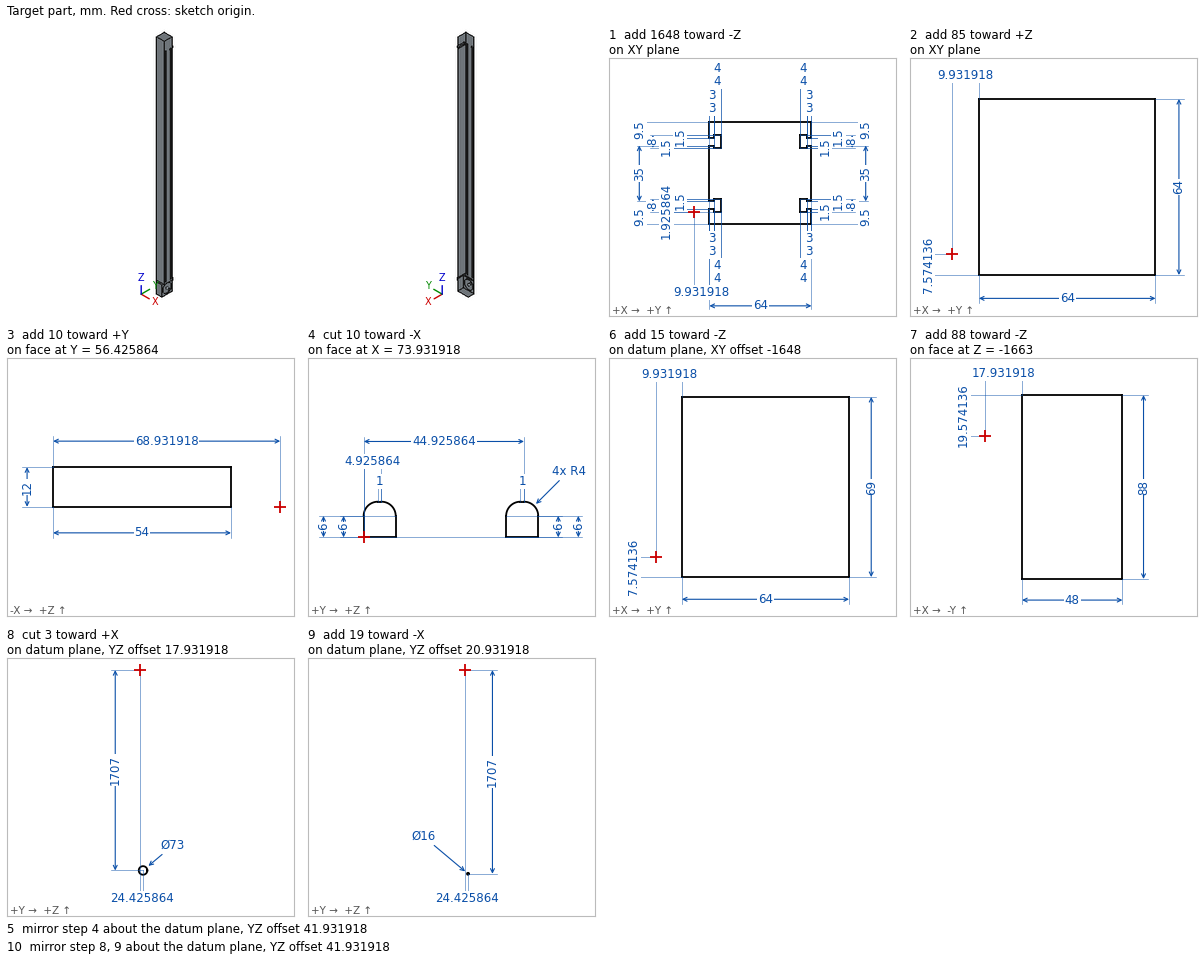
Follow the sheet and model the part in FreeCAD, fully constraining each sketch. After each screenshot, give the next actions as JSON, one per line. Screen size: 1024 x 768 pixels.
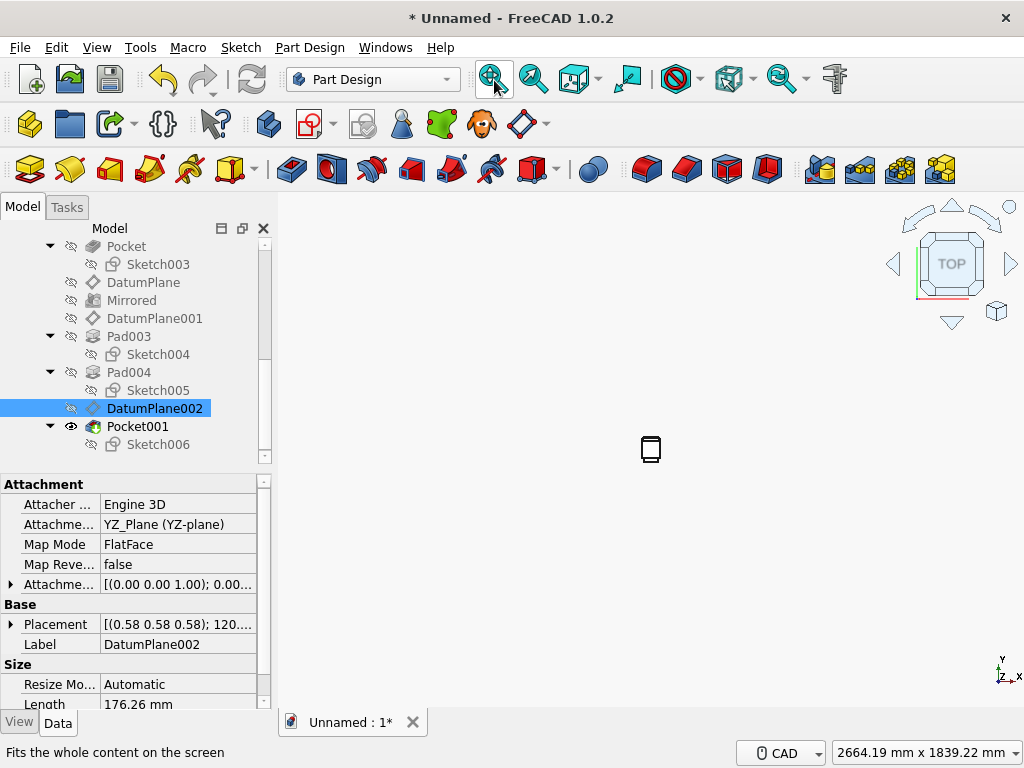
{"action": "key", "text": "1"}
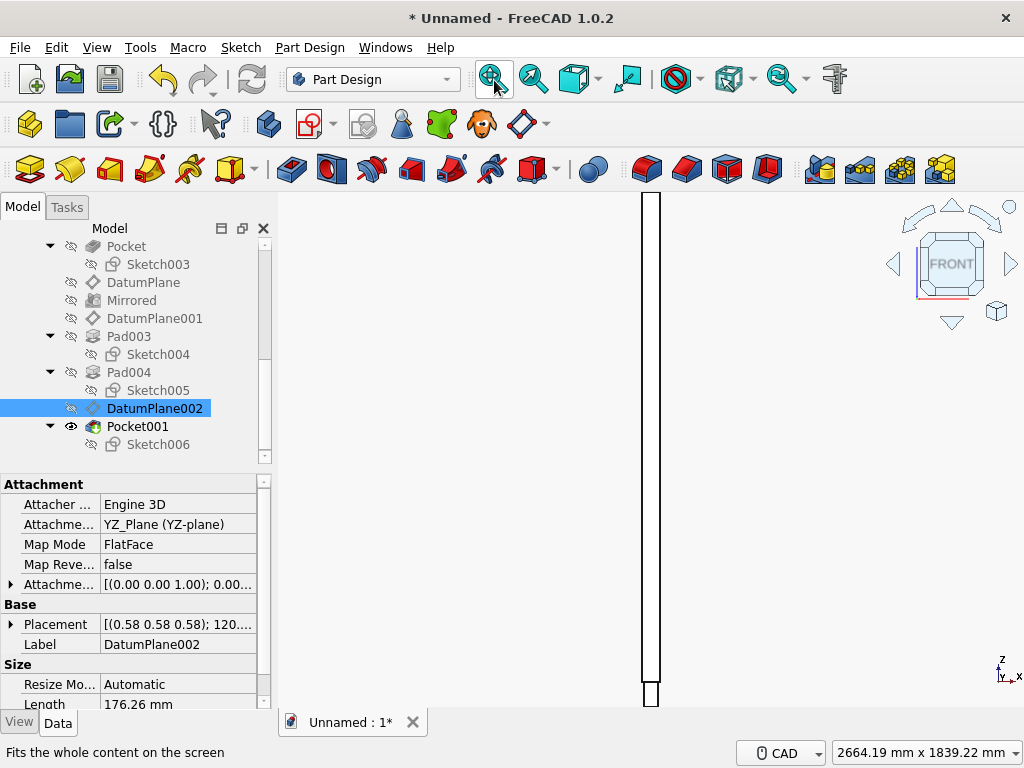
{"action": "left_click", "coordinate": [494, 80]}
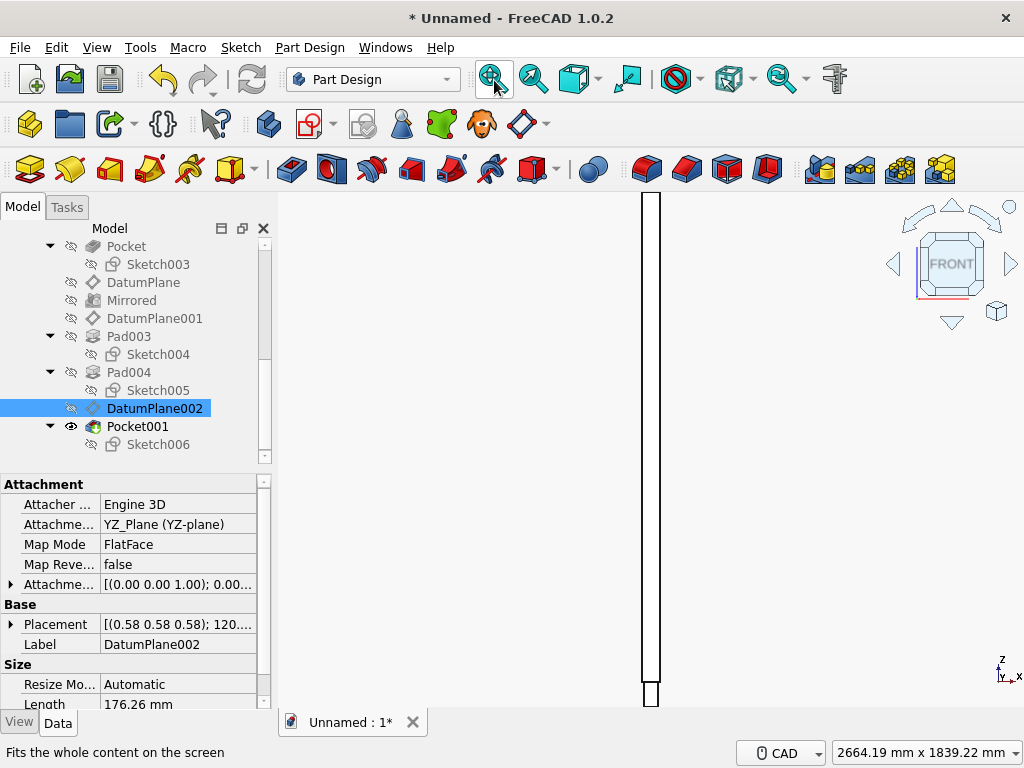
{"action": "scroll", "coordinate": [140, 350], "scroll_direction": "down", "scroll_amount": 3}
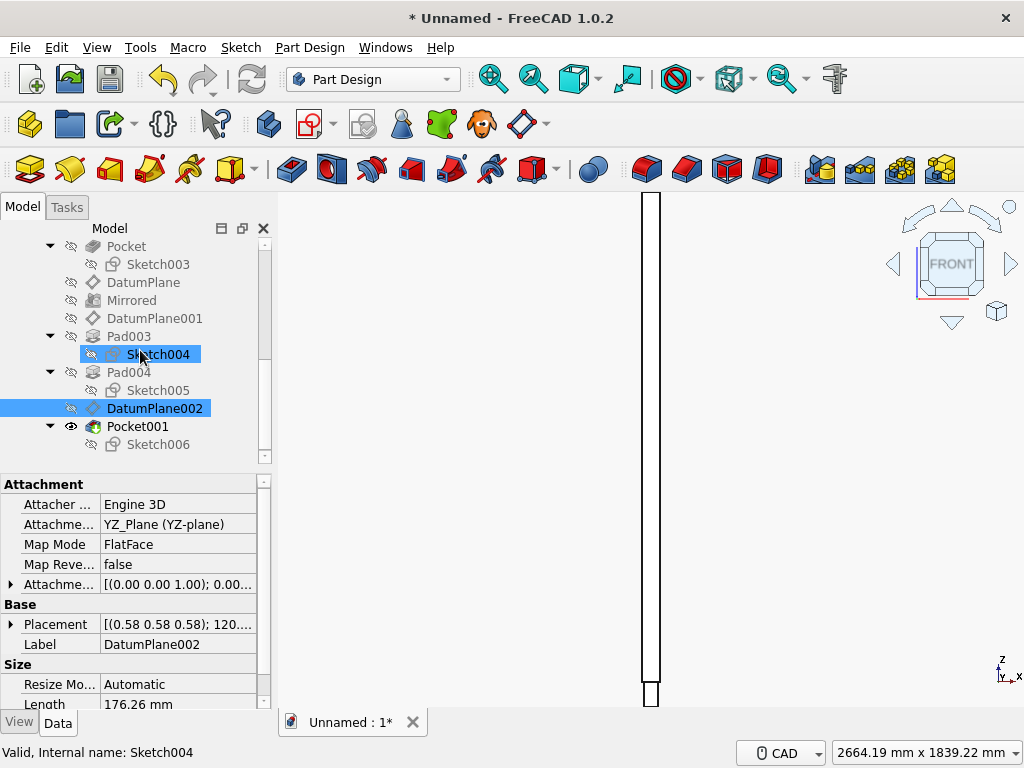
{"action": "scroll", "coordinate": [140, 350], "scroll_direction": "up", "scroll_amount": 15}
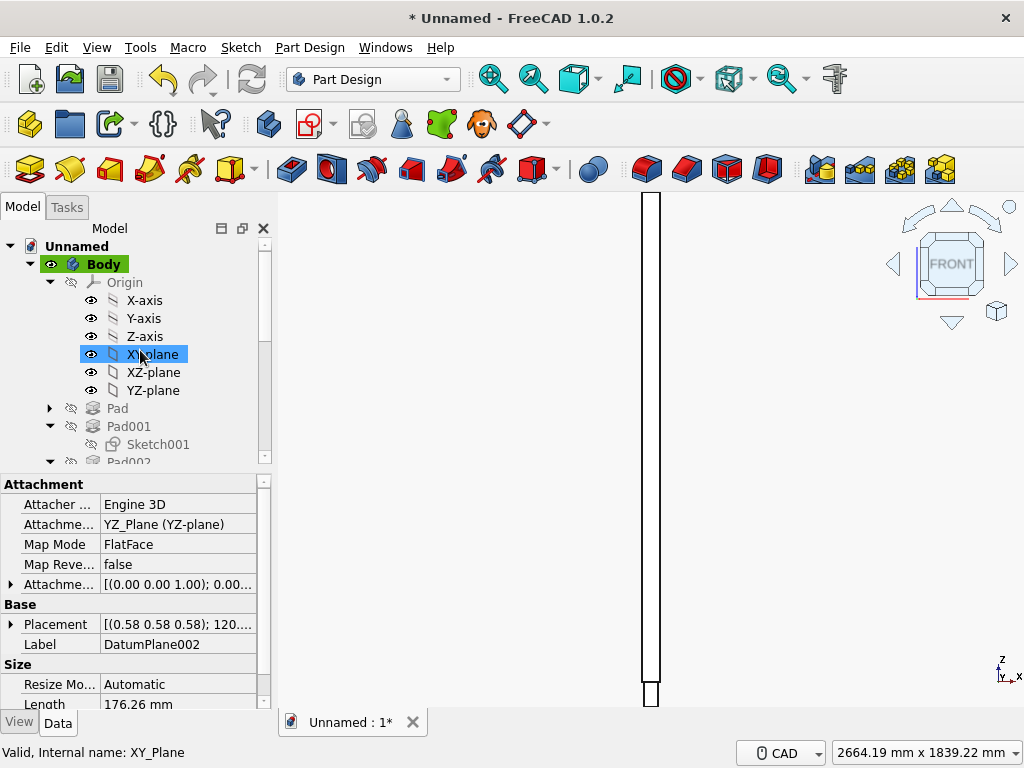
{"action": "left_click", "coordinate": [136, 390]}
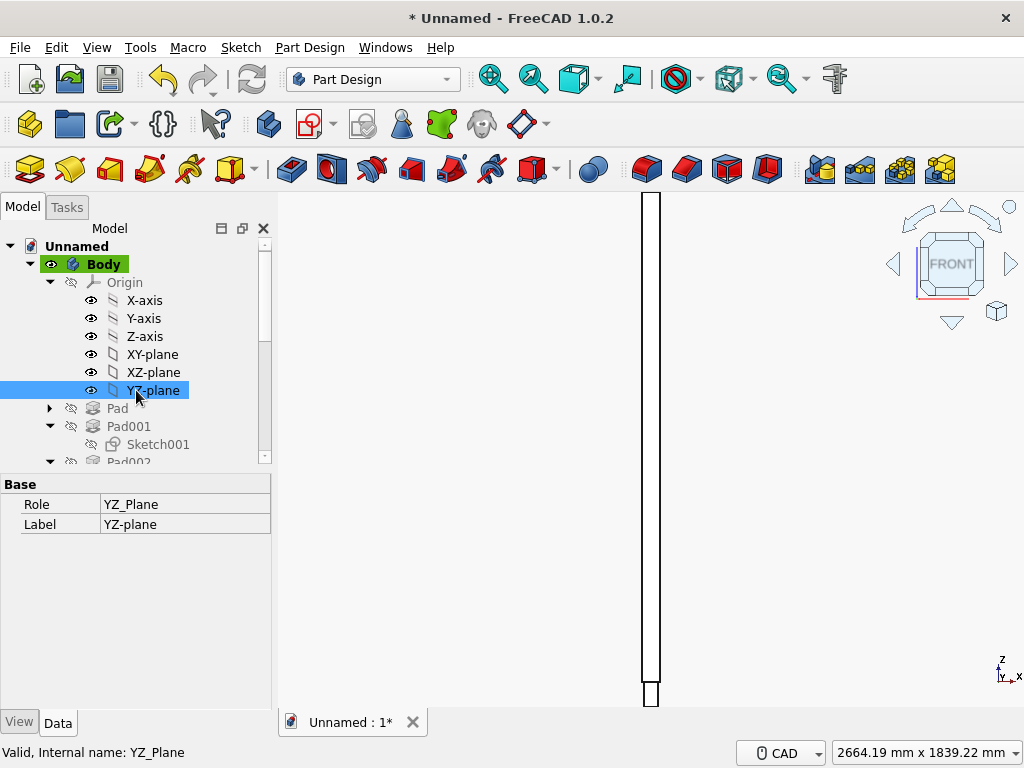
{"action": "left_click", "coordinate": [522, 124]}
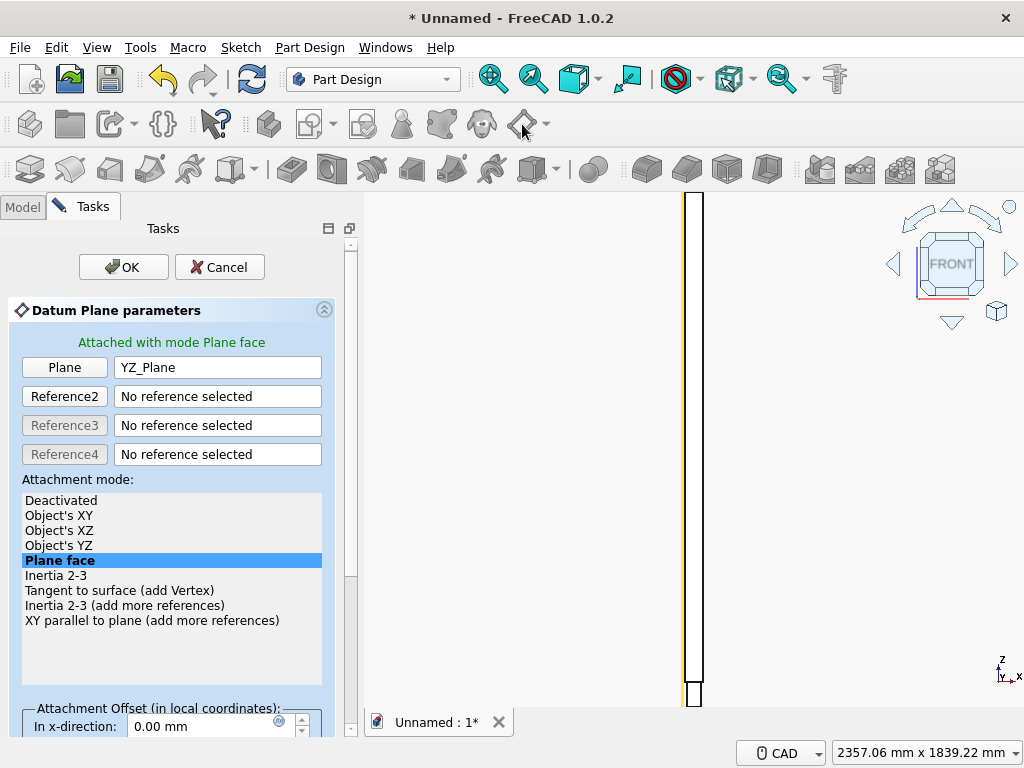
{"action": "scroll", "coordinate": [351, 487], "scroll_direction": "down", "scroll_amount": 3}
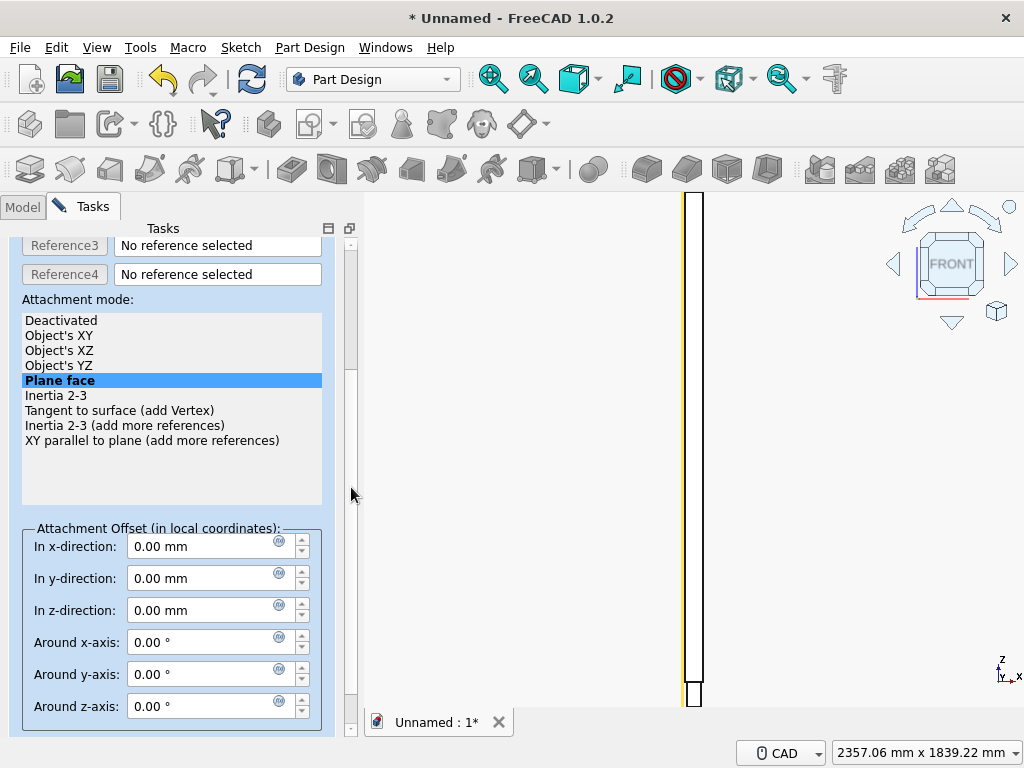
{"action": "triple_click", "coordinate": [210, 610]}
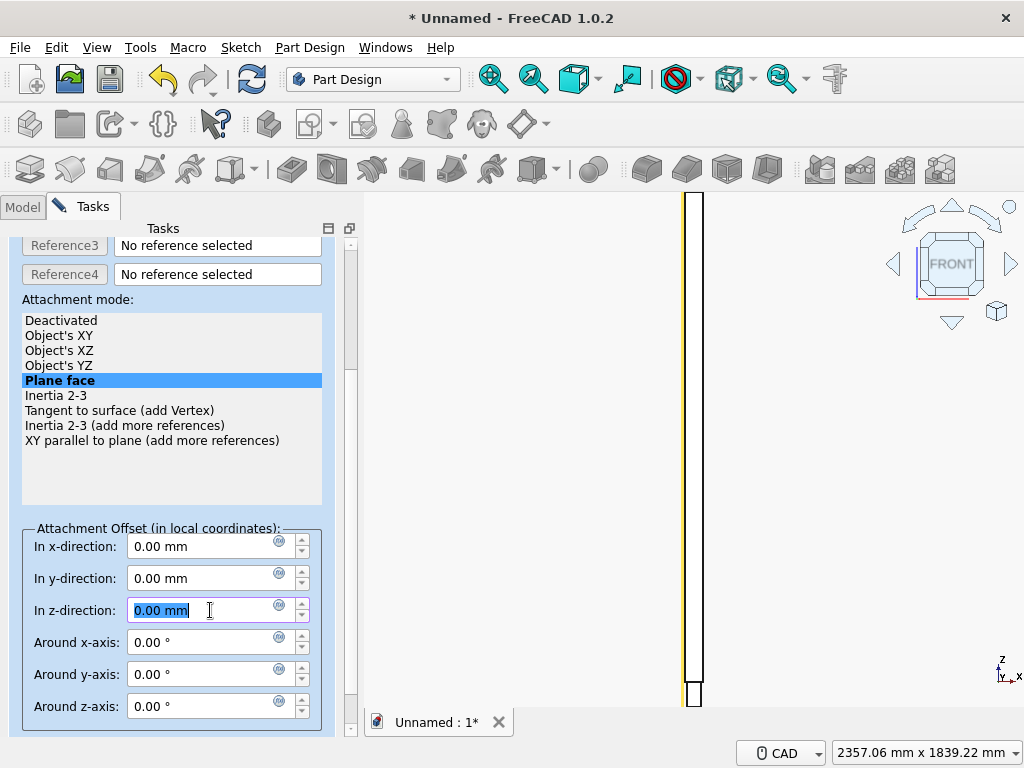
{"action": "type", "text": "20.931918"}
{"action": "key", "text": "Tab"}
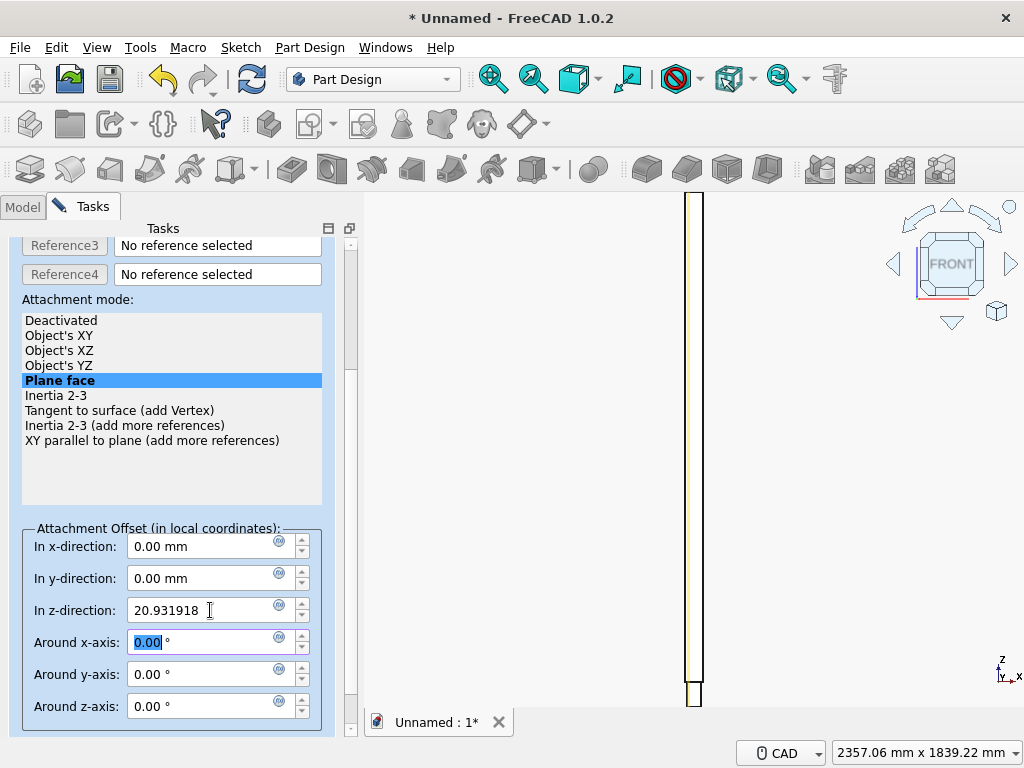
{"action": "scroll", "coordinate": [351, 487], "scroll_direction": "up", "scroll_amount": 4}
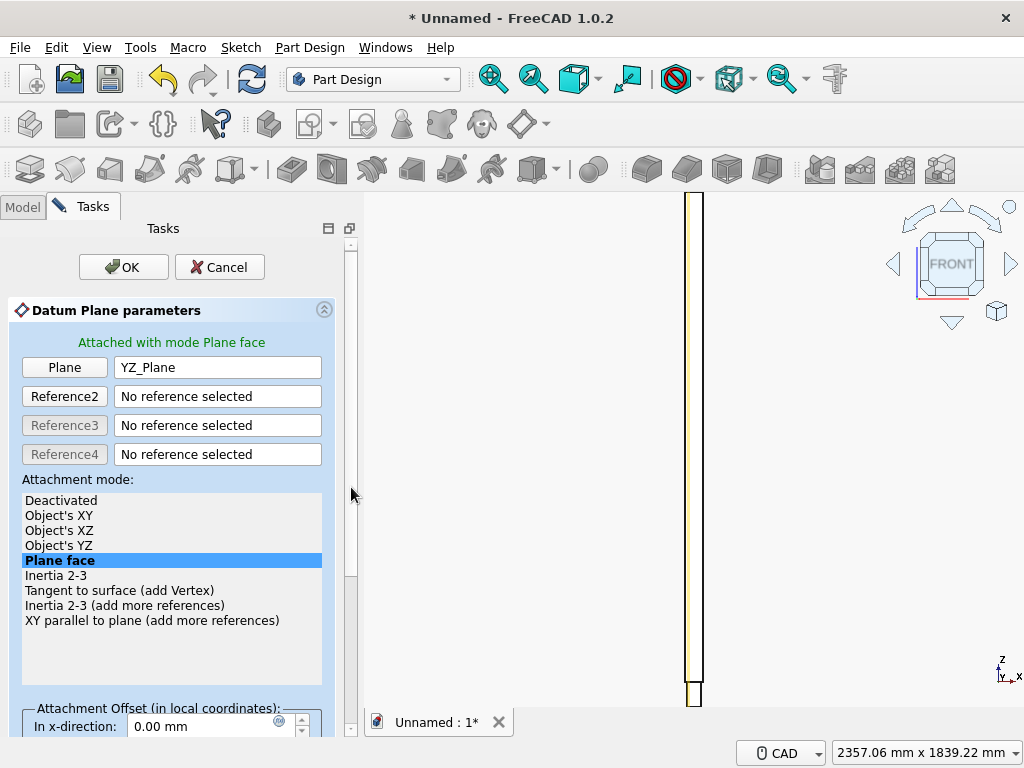
{"action": "left_click", "coordinate": [124, 267]}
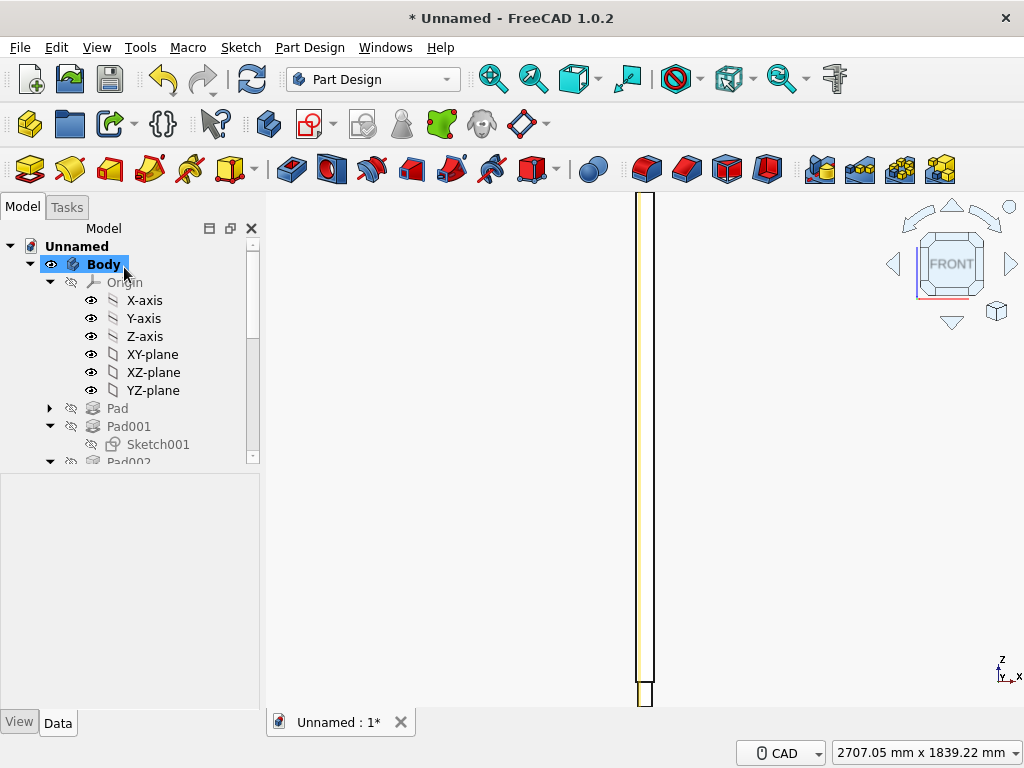
{"action": "scroll", "coordinate": [100, 350], "scroll_direction": "down", "scroll_amount": 3}